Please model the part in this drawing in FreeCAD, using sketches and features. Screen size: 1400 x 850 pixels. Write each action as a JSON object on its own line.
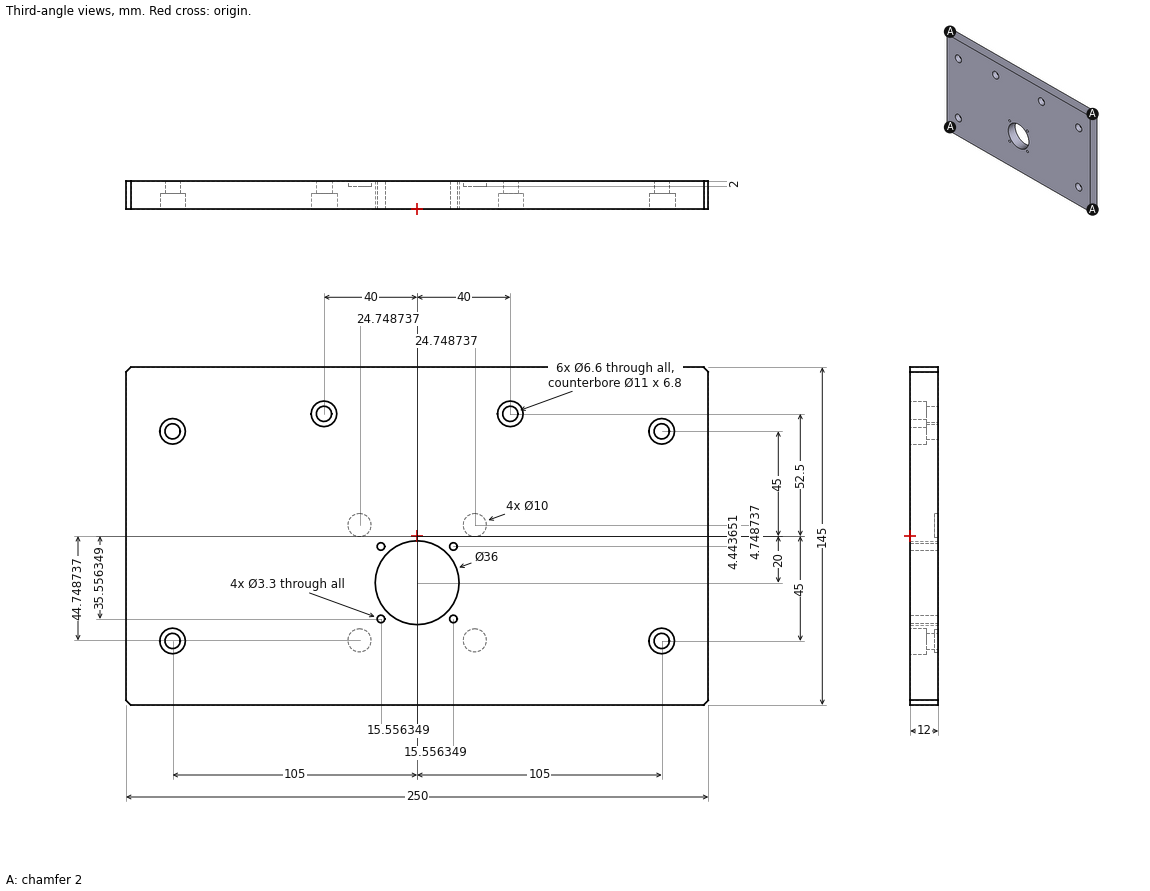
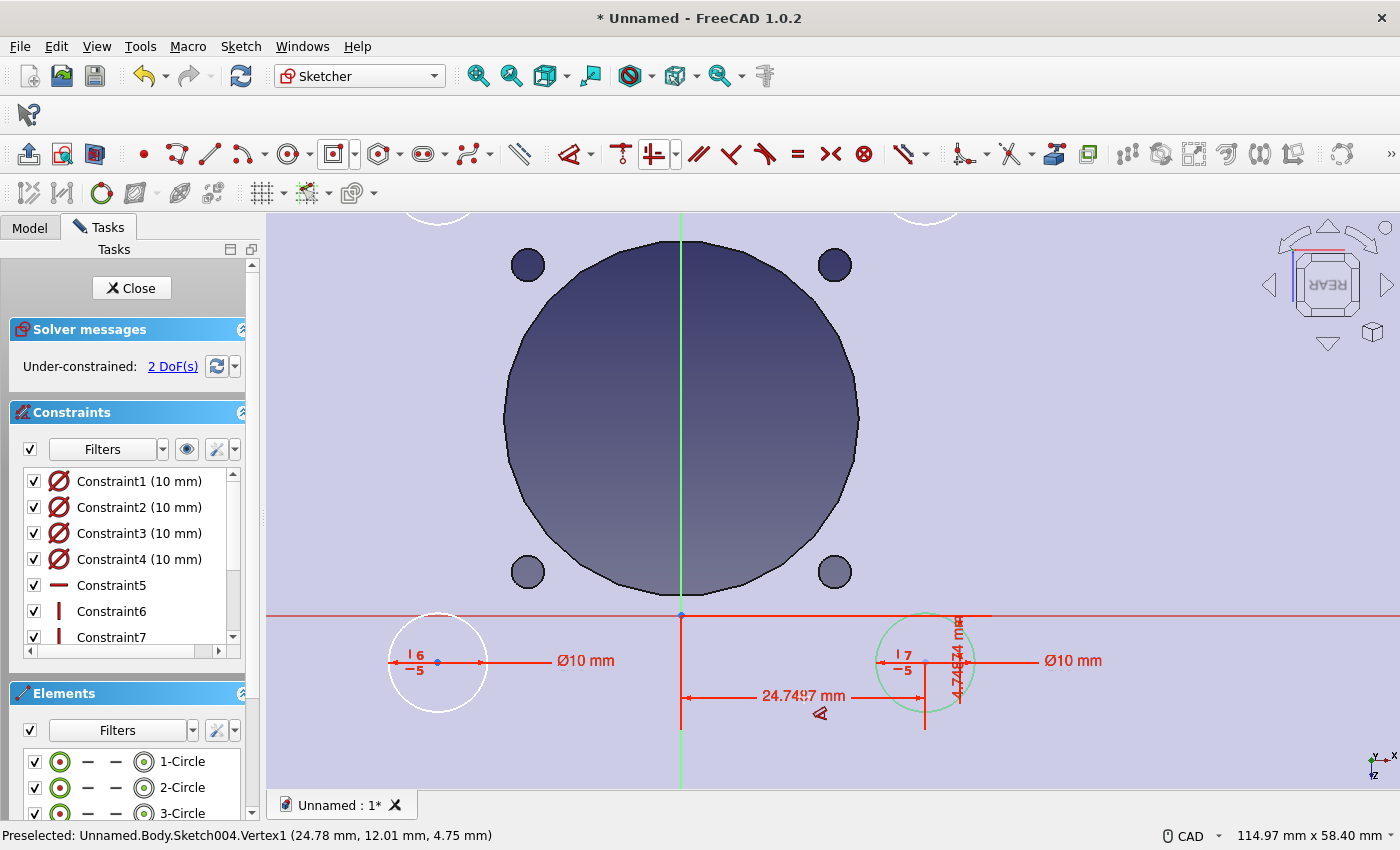
{"action": "left_click", "coordinate": [438, 663]}
{"action": "left_click", "coordinate": [560, 697]}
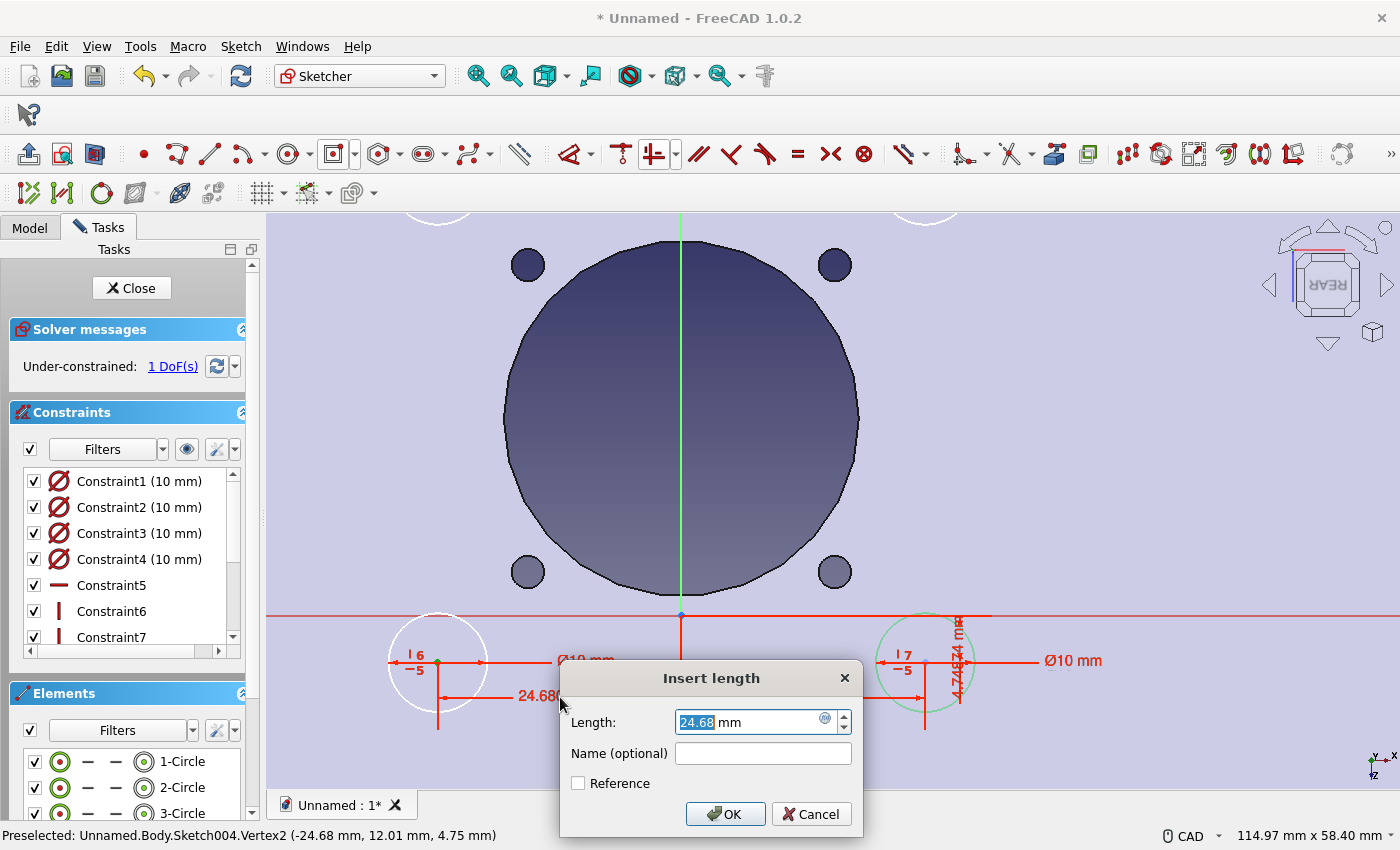
{"action": "type", "text": "24.748737"}
{"action": "key", "text": "Return"}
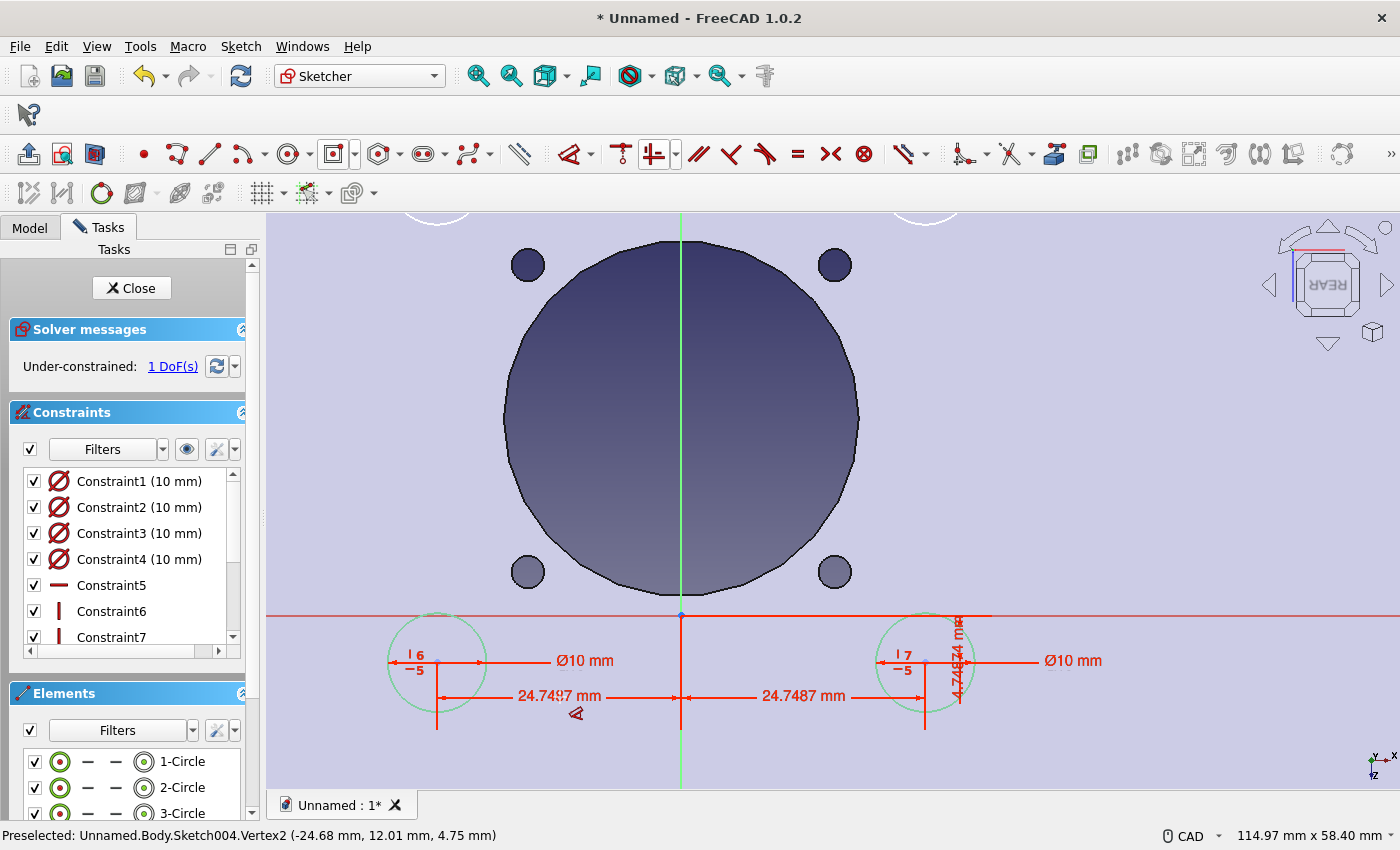
{"action": "scroll", "coordinate": [934, 669], "scroll_direction": "down", "scroll_amount": 2}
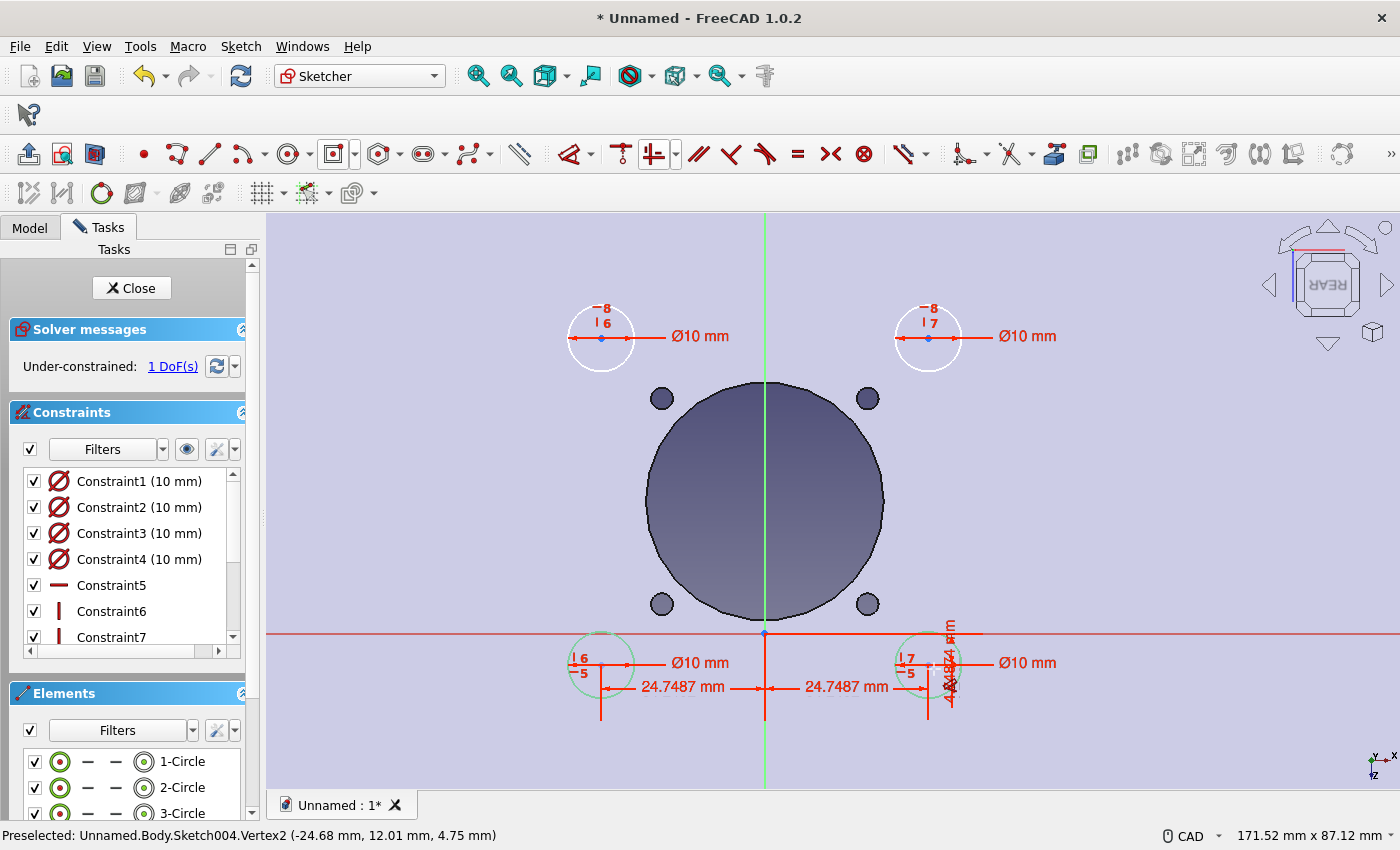
{"action": "left_click", "coordinate": [601, 338]}
{"action": "left_click", "coordinate": [567, 486]}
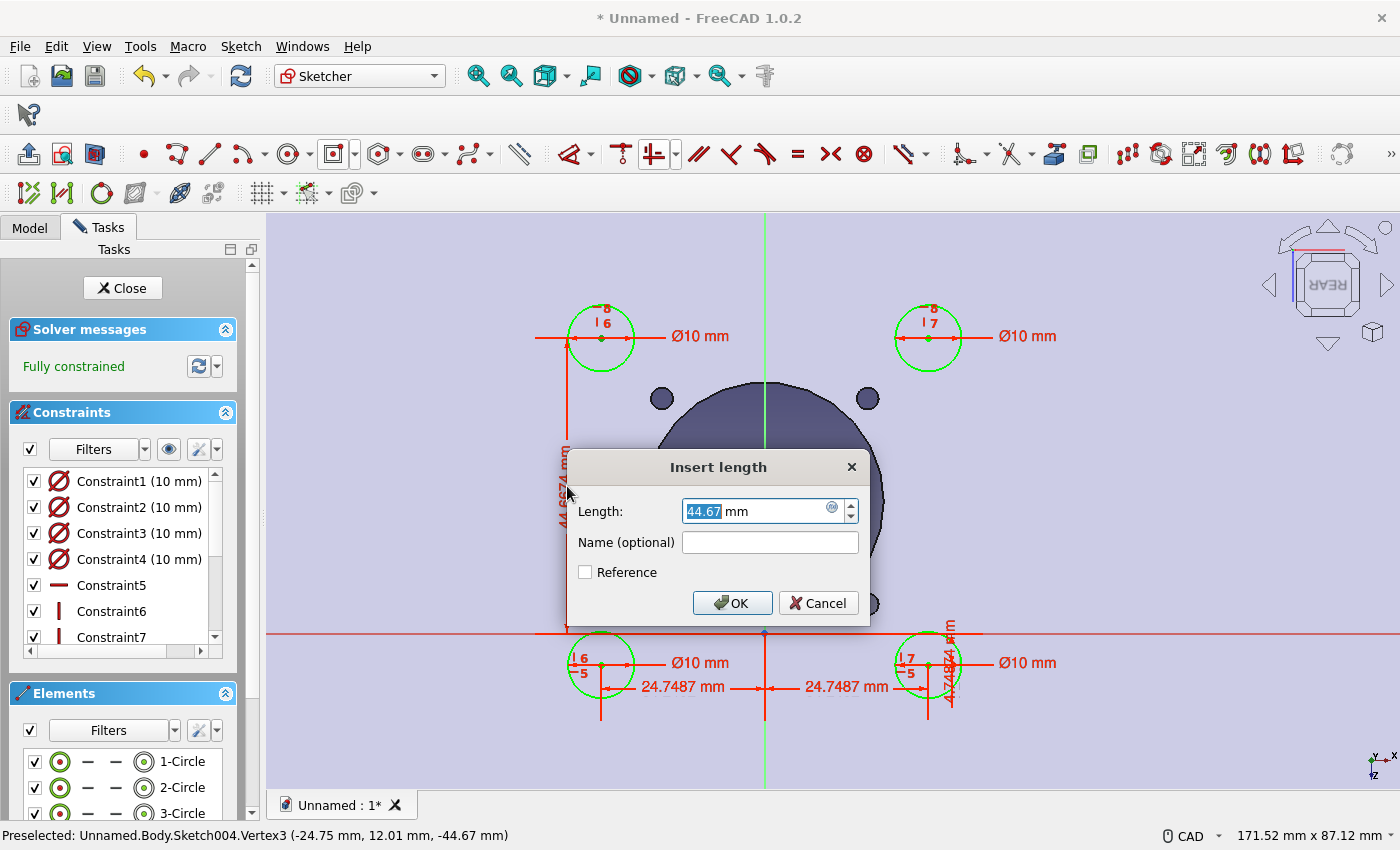
{"action": "type", "text": "44.748737"}
{"action": "key", "text": "Return"}
{"action": "key", "text": "Escape"}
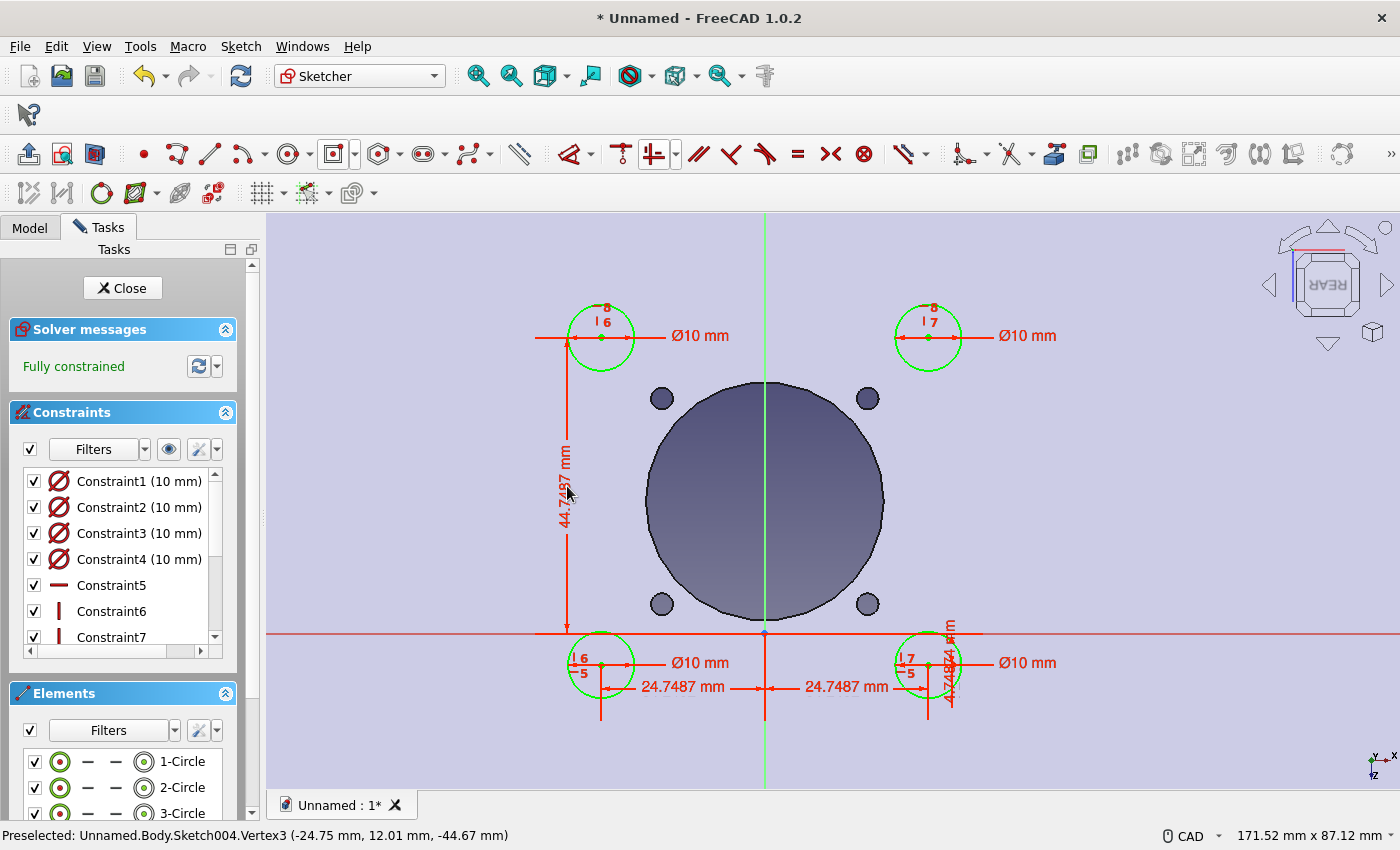
{"action": "left_click", "coordinate": [123, 288]}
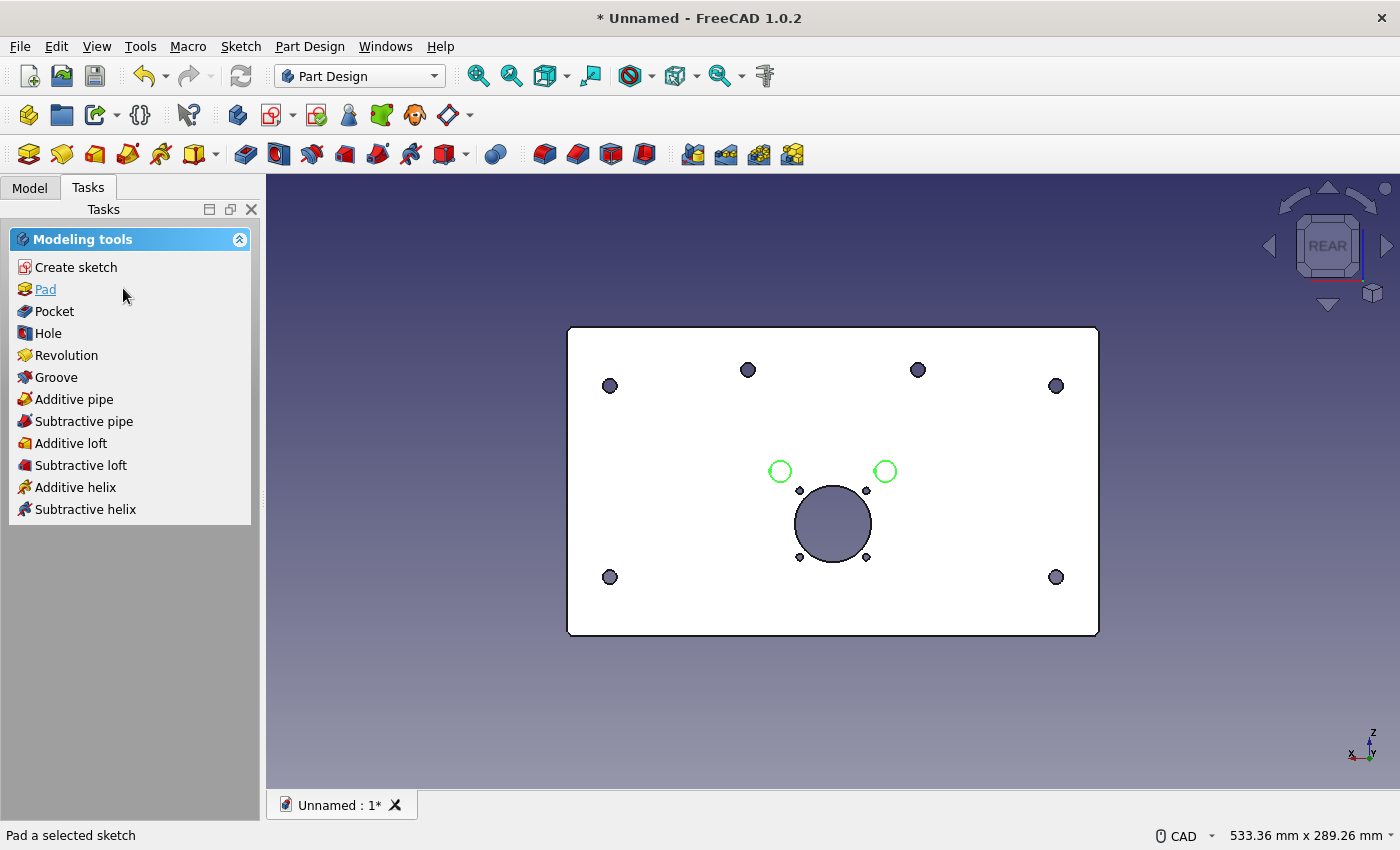
{"action": "left_click", "coordinate": [246, 154]}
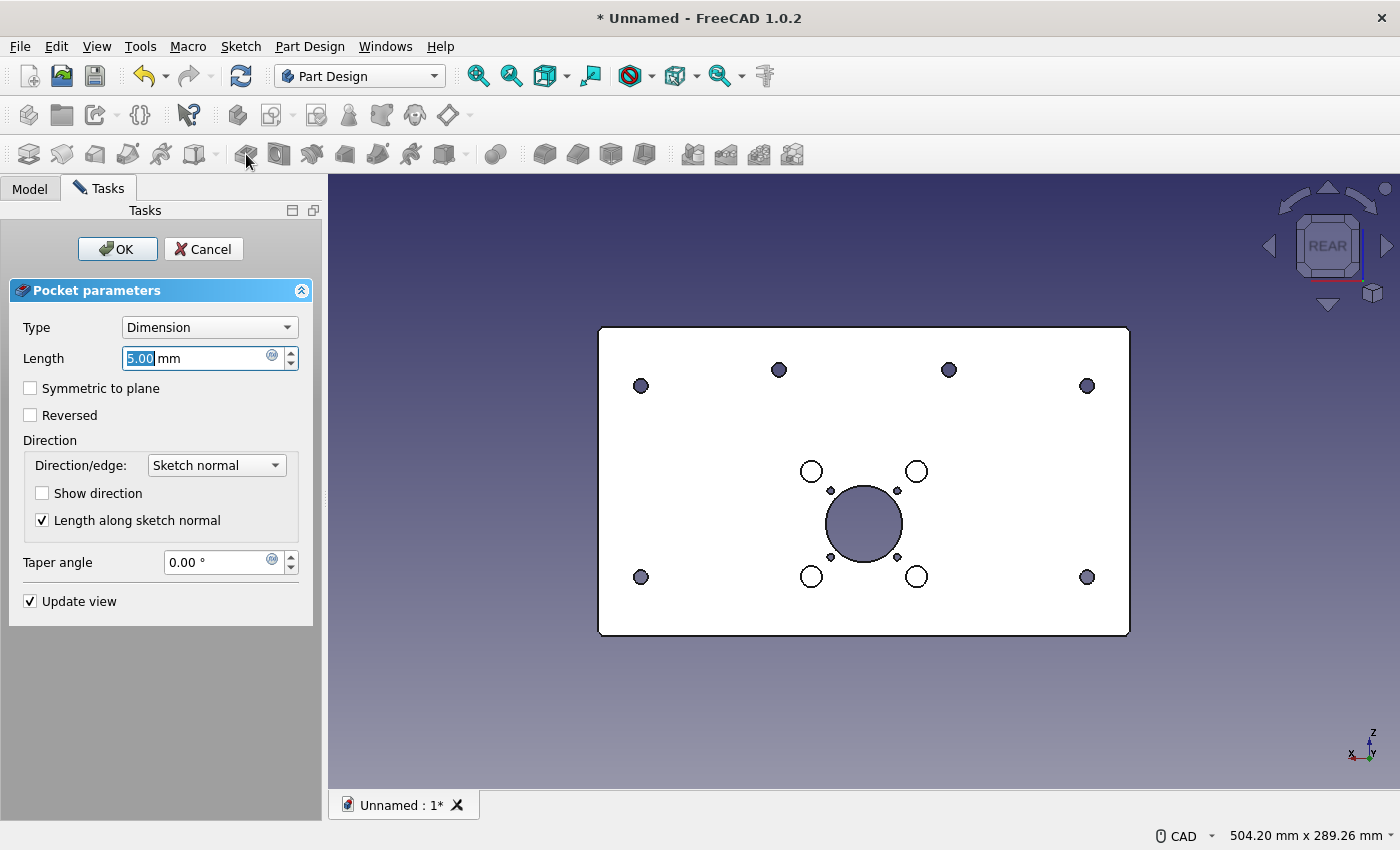
{"action": "type", "text": "2"}
{"action": "key", "text": "Tab"}